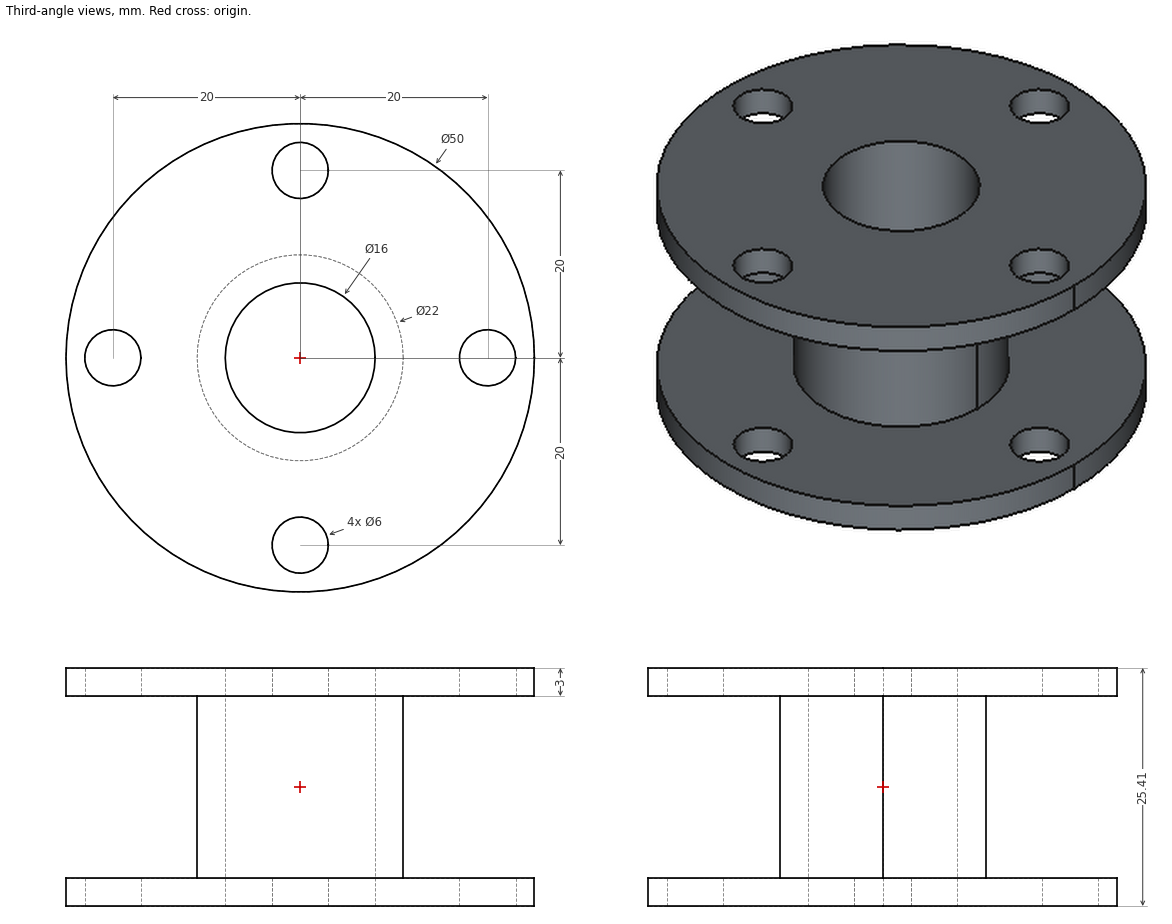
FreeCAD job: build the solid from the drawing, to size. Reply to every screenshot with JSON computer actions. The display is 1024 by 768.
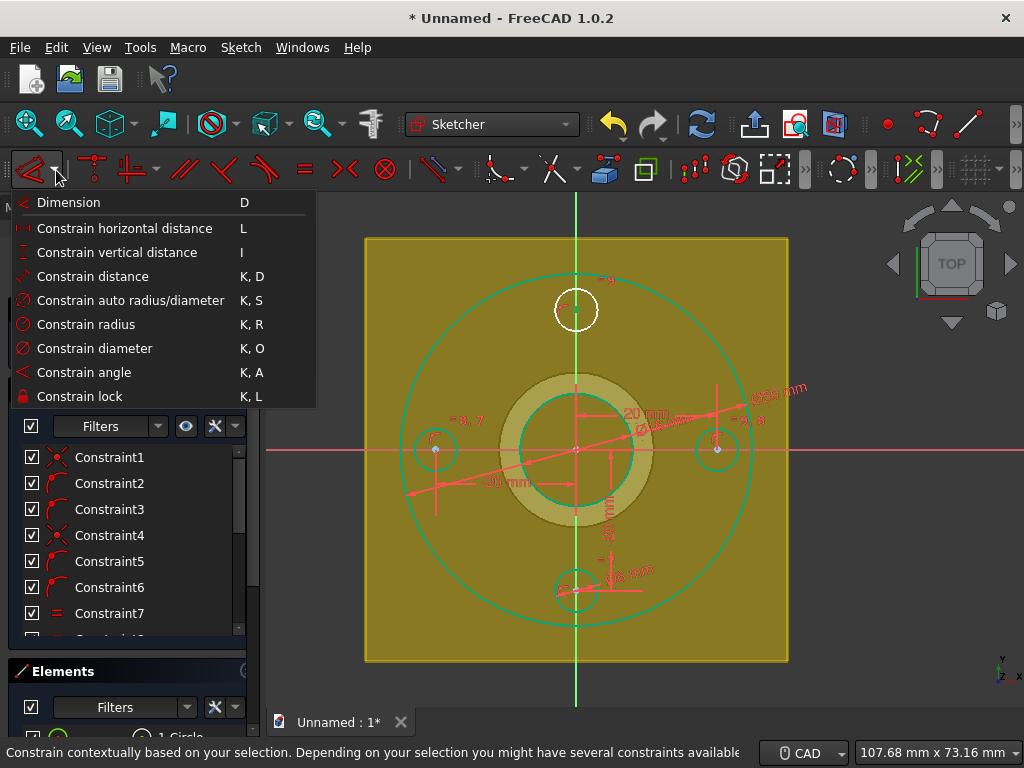
{"action": "left_click", "coordinate": [164, 252]}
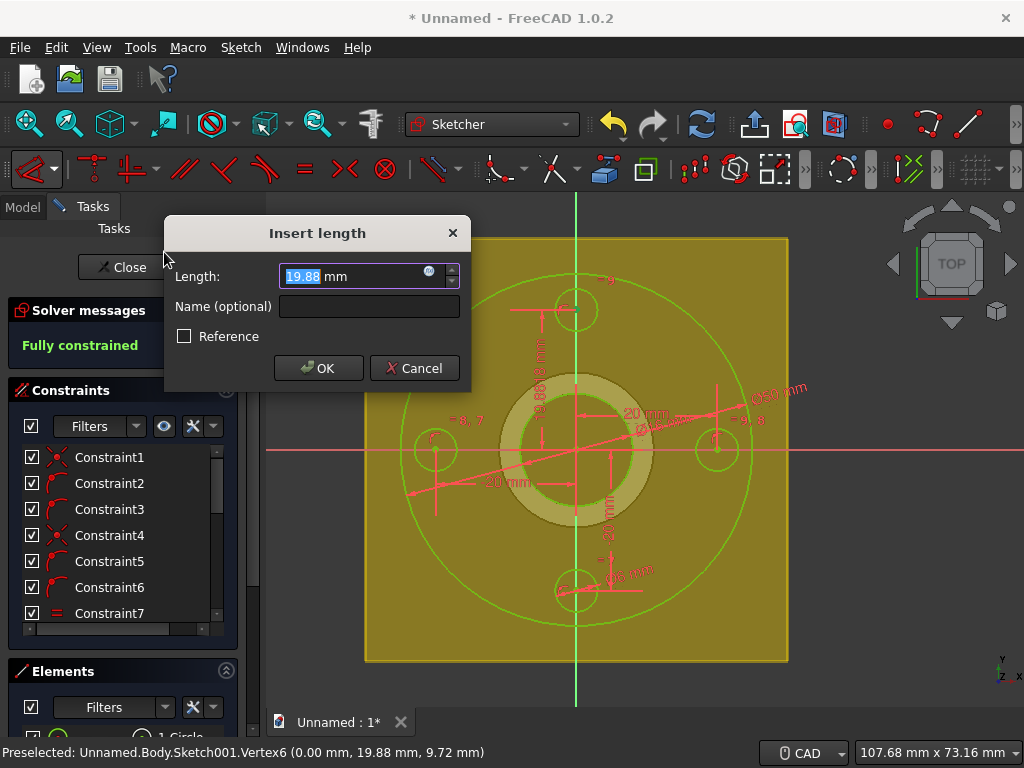
{"action": "type", "text": "20"}
{"action": "key", "text": "Return"}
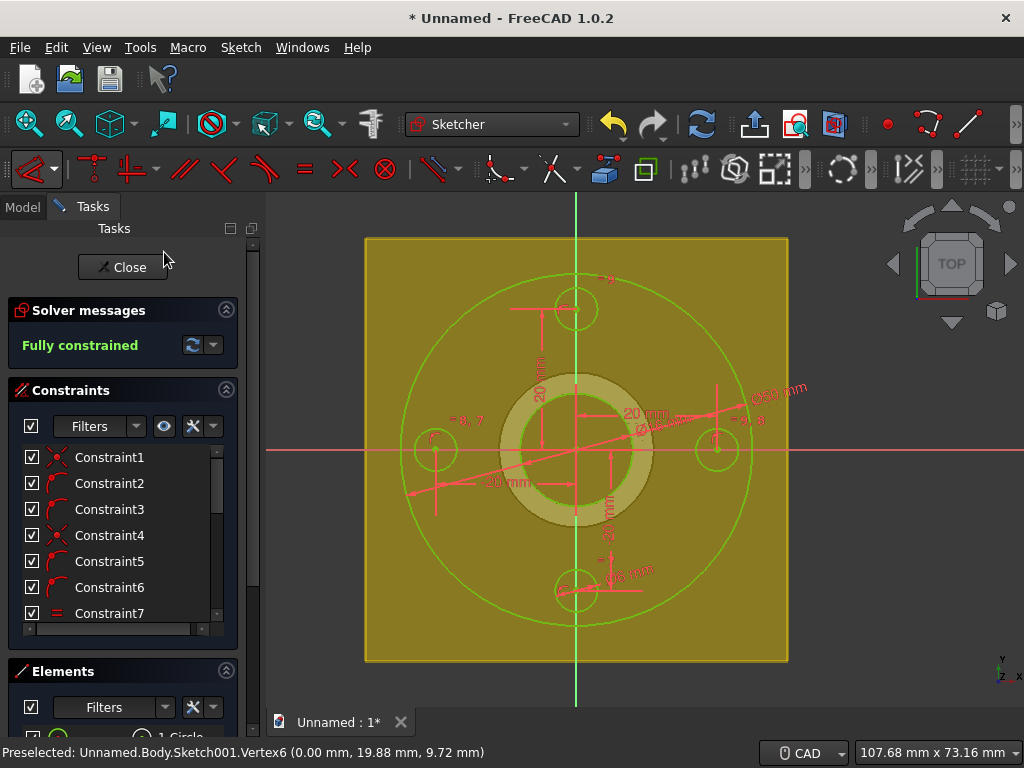
{"action": "left_click", "coordinate": [123, 267]}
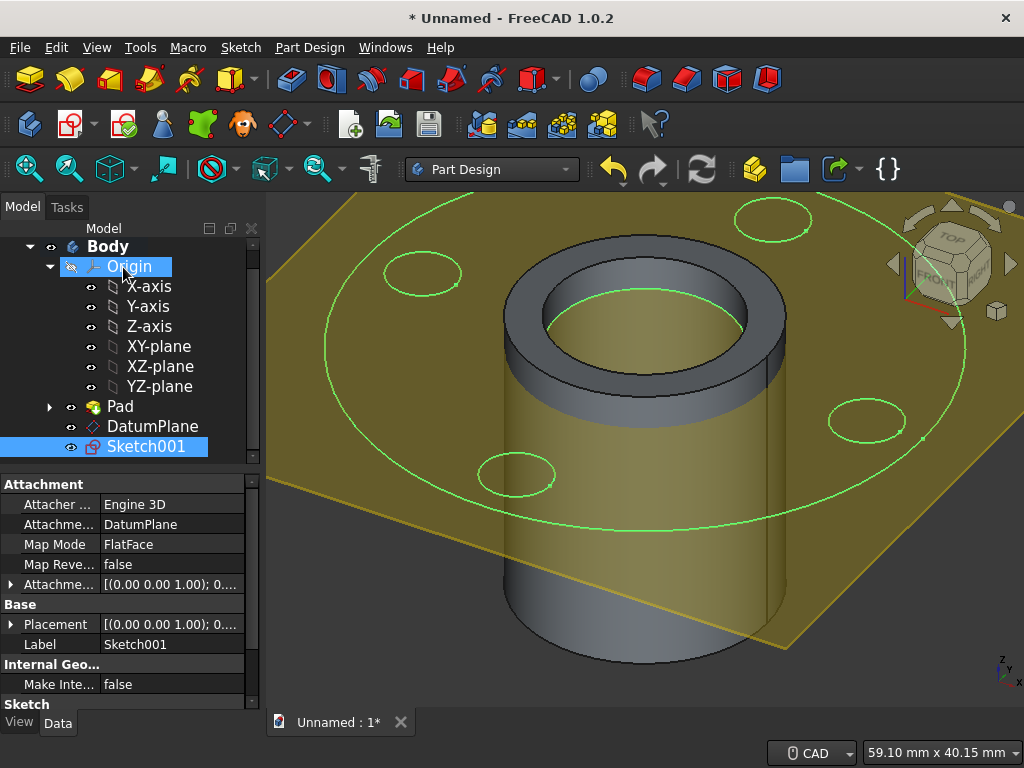
{"action": "left_click", "coordinate": [30, 80]}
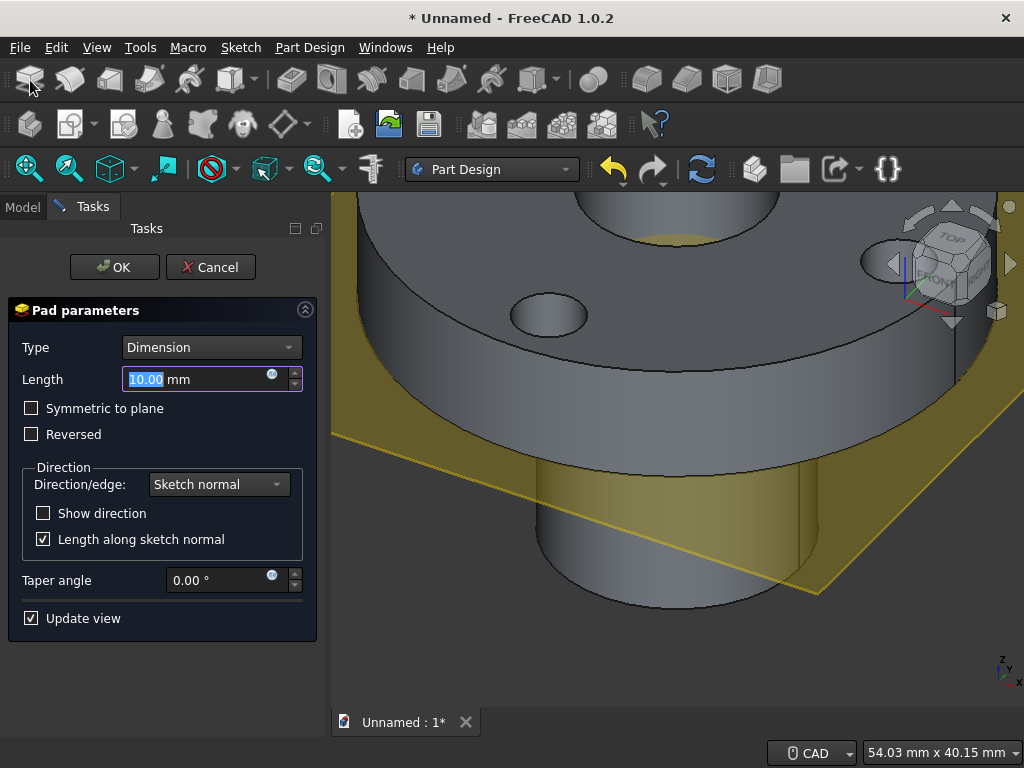
{"action": "type", "text": "3"}
{"action": "key", "text": "Tab"}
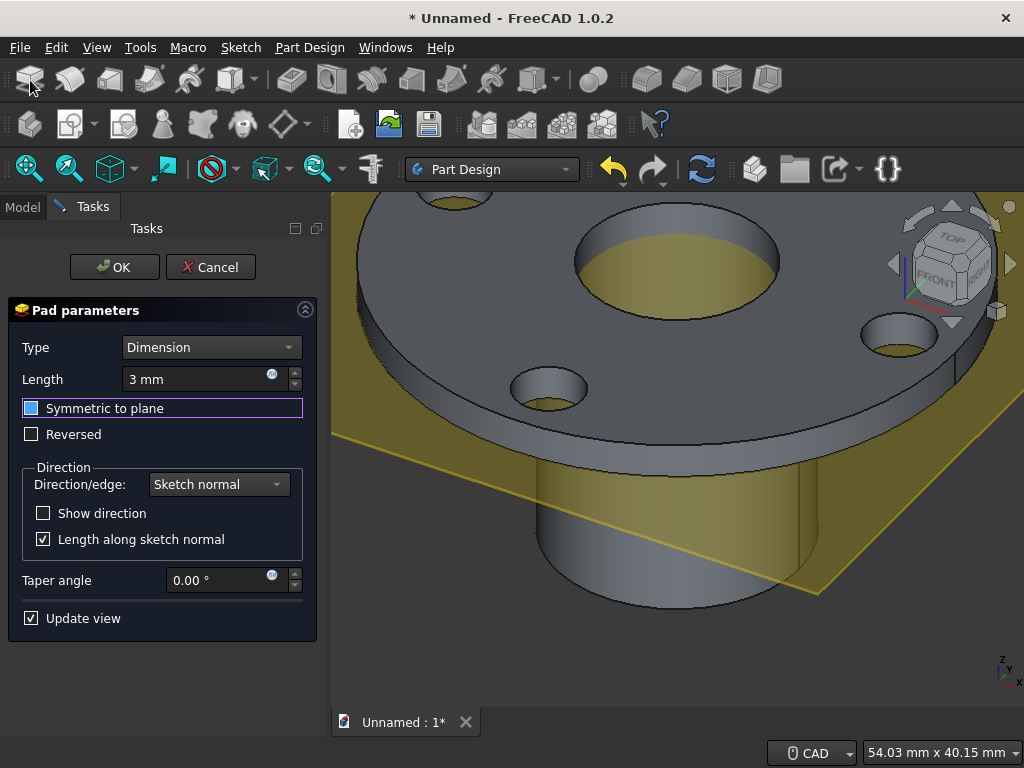
{"action": "left_click", "coordinate": [115, 267]}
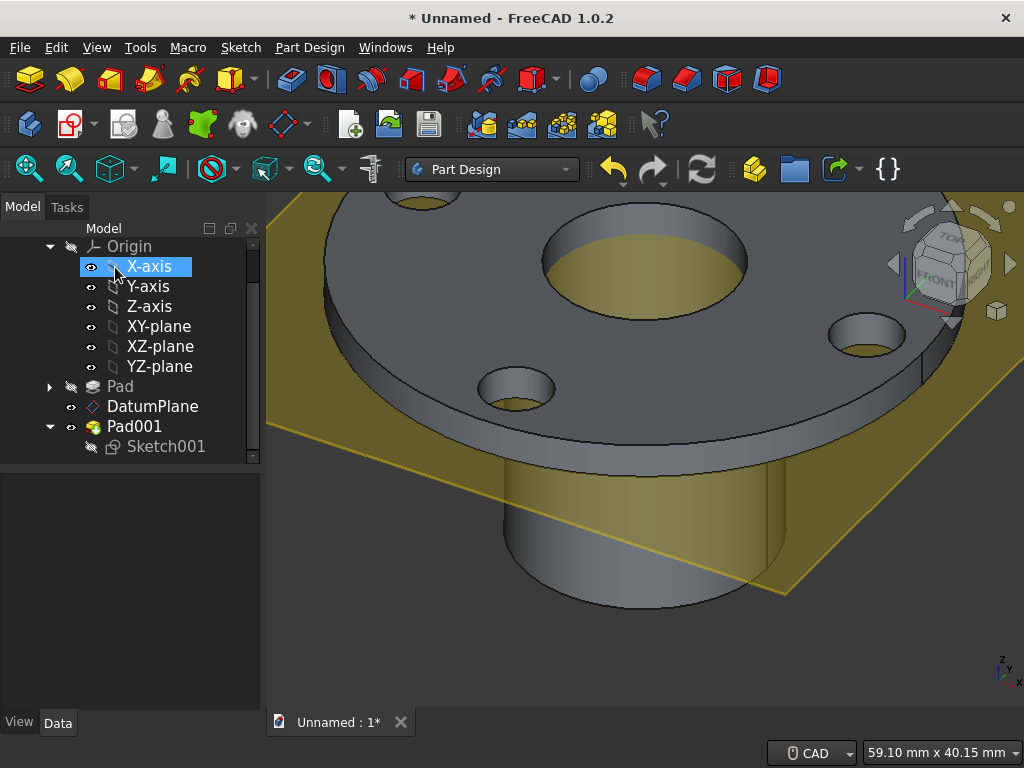
{"action": "left_click", "coordinate": [116, 407]}
{"action": "key", "text": "space"}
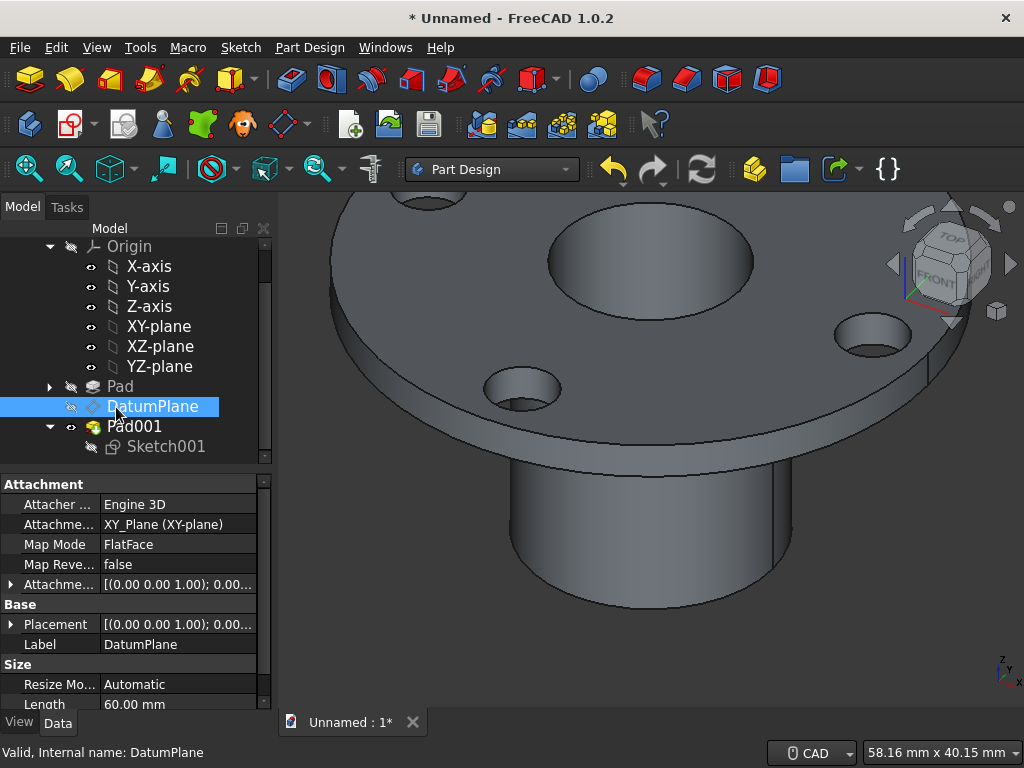
{"action": "left_click", "coordinate": [30, 170]}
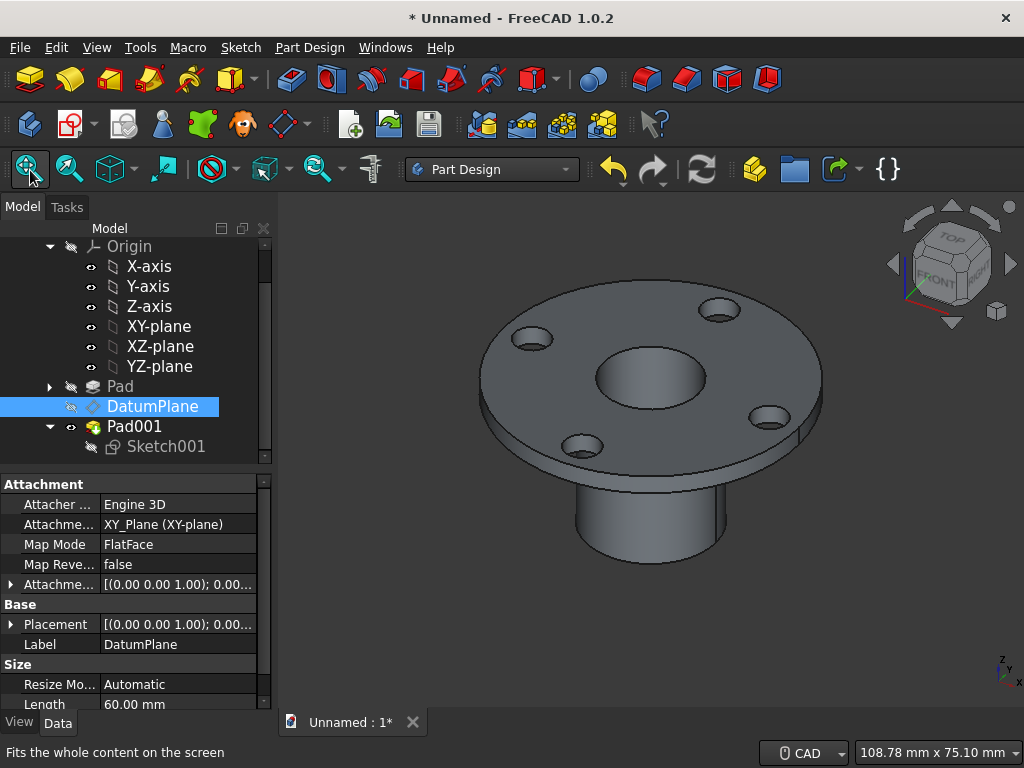
{"action": "left_click", "coordinate": [116, 427]}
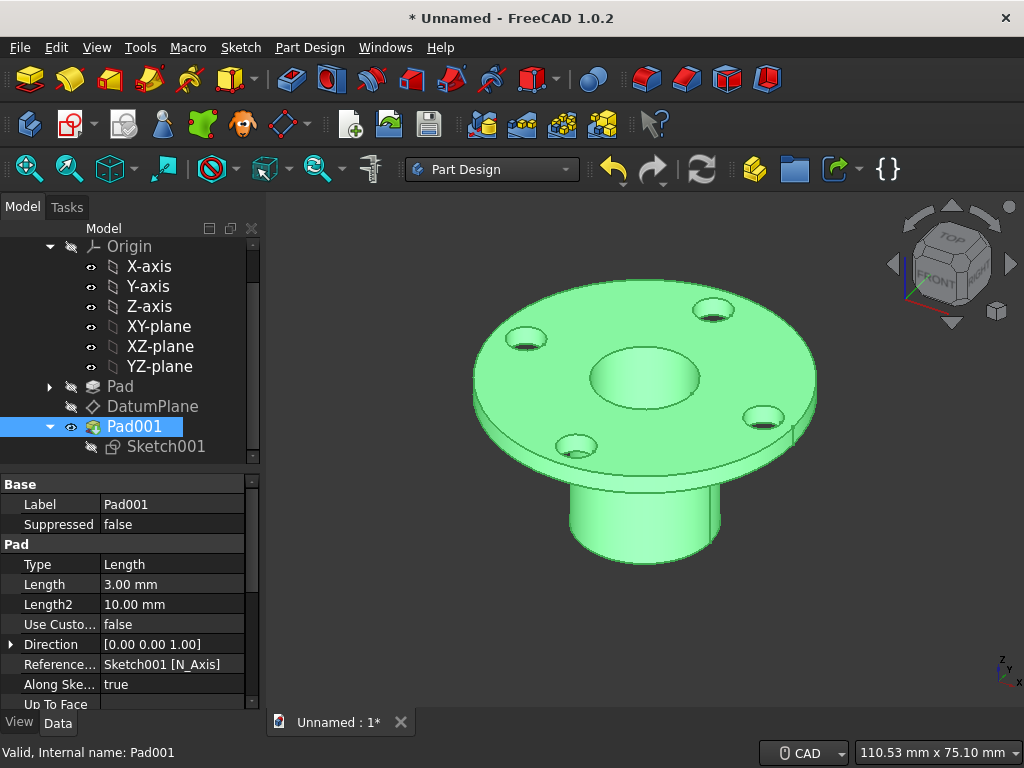
{"action": "left_click", "coordinate": [482, 124]}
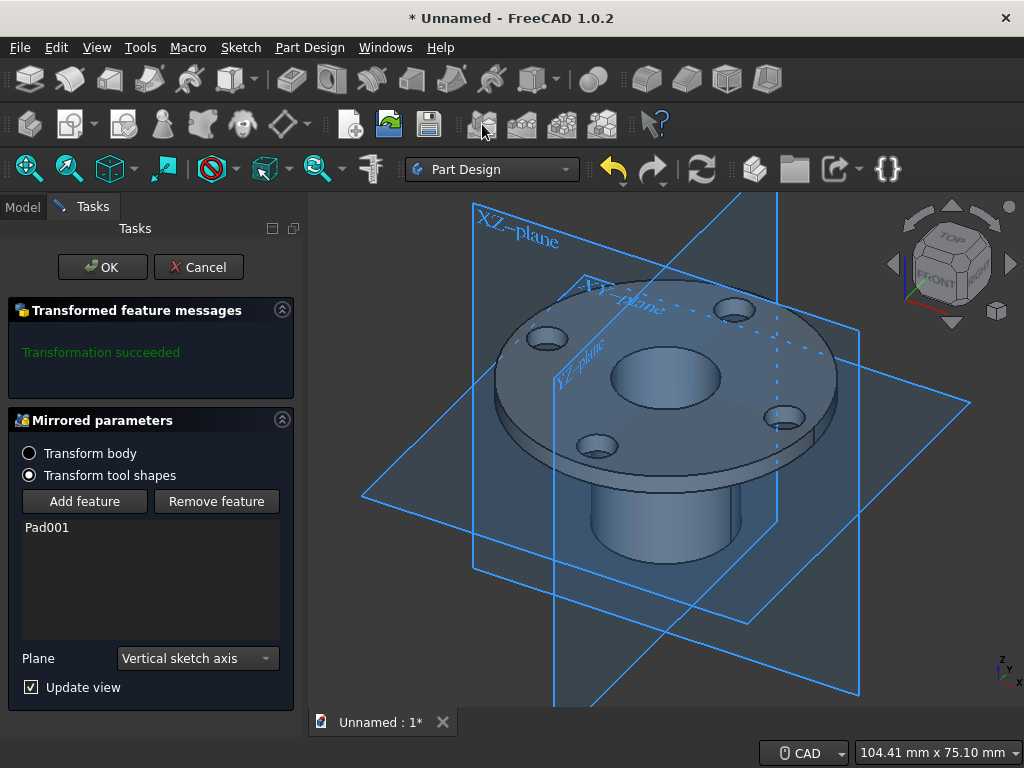
{"action": "left_click", "coordinate": [198, 658]}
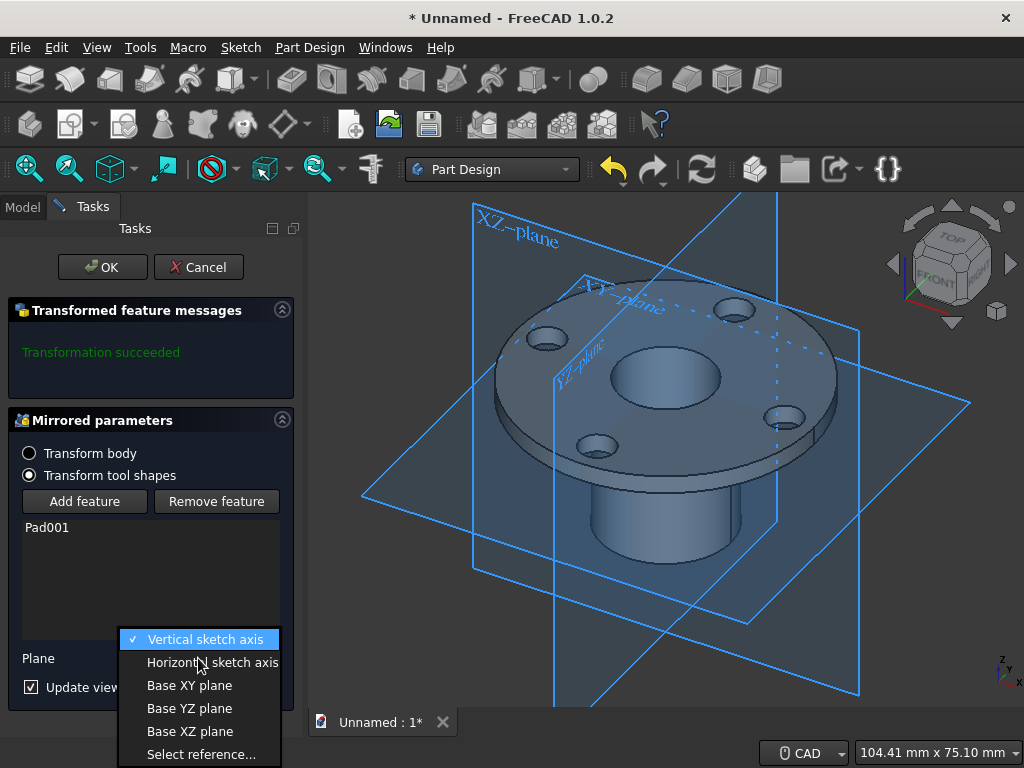
{"action": "left_click", "coordinate": [198, 686]}